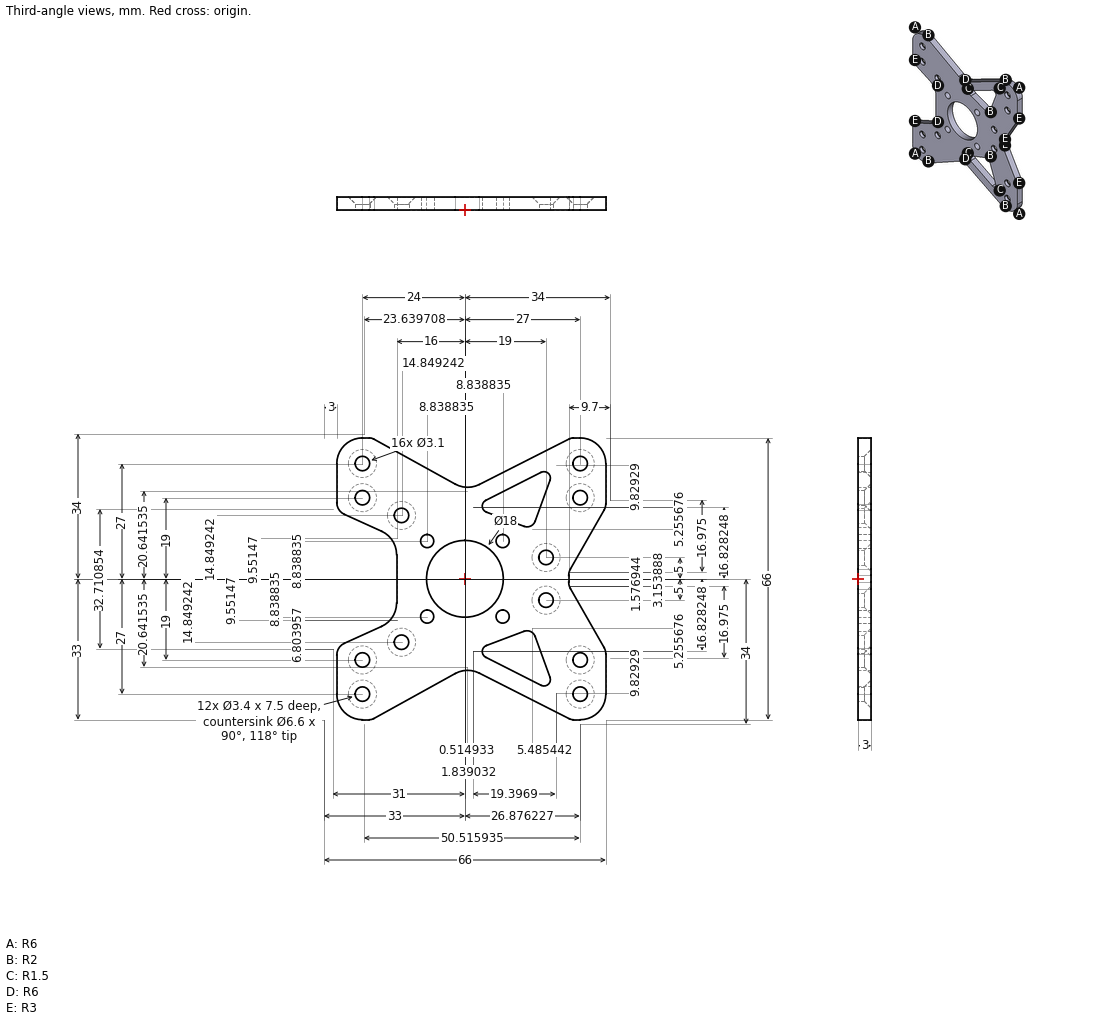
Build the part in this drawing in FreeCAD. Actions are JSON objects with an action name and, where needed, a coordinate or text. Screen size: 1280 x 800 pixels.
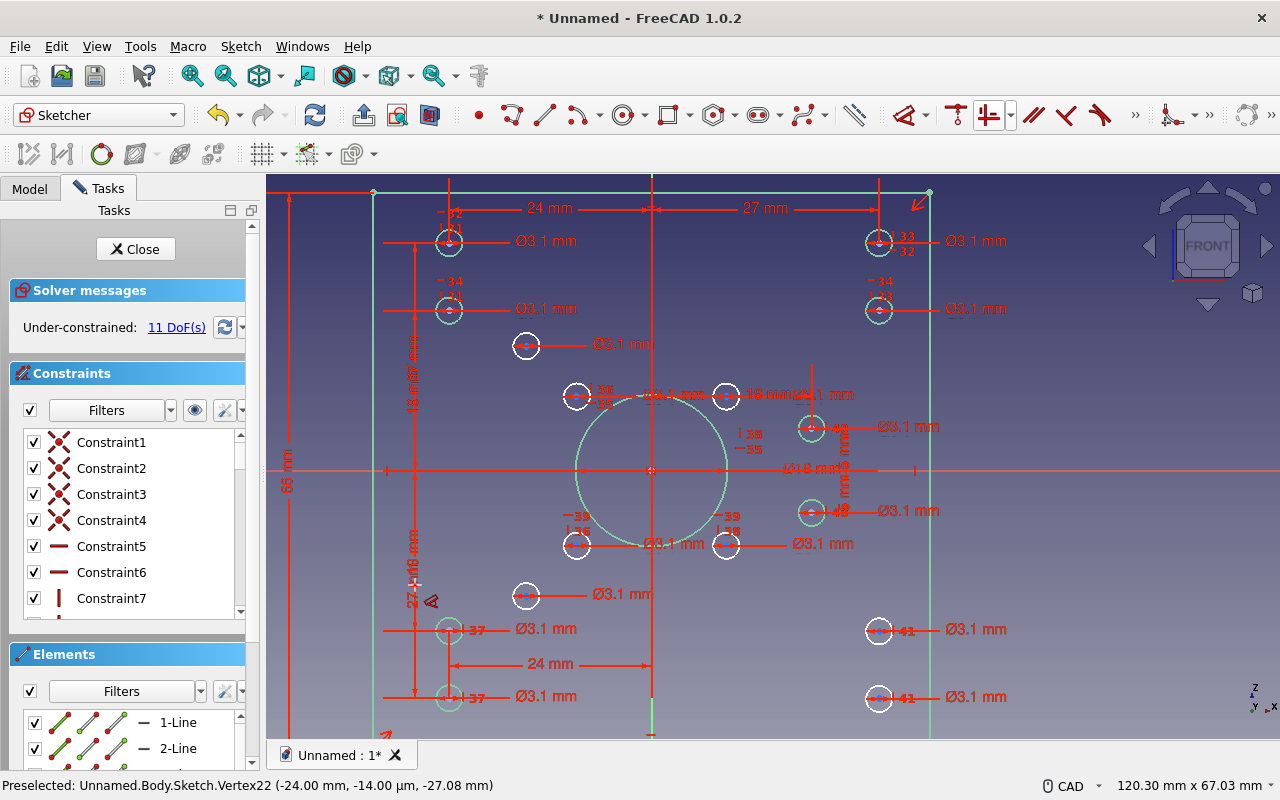
{"action": "left_click", "coordinate": [879, 631]}
{"action": "left_click", "coordinate": [765, 665]}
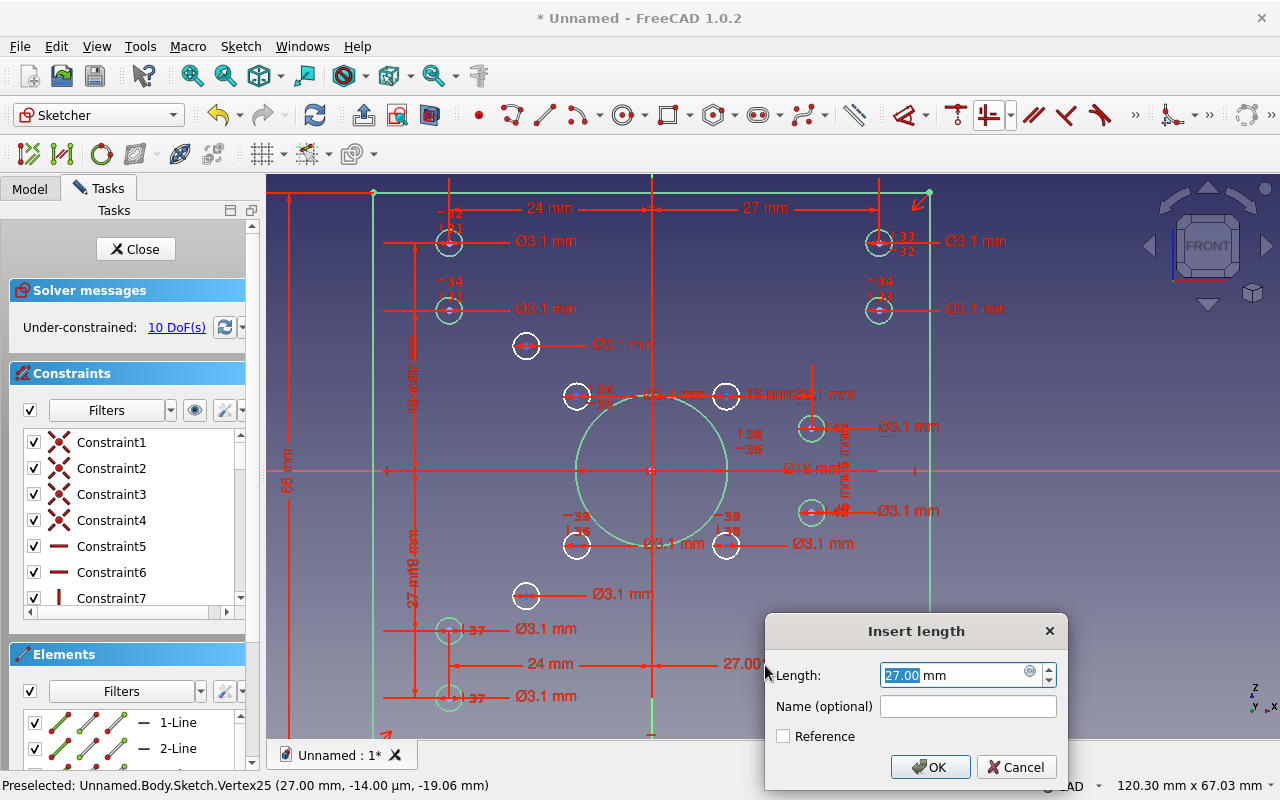
{"action": "type", "text": "27"}
{"action": "key", "text": "Return"}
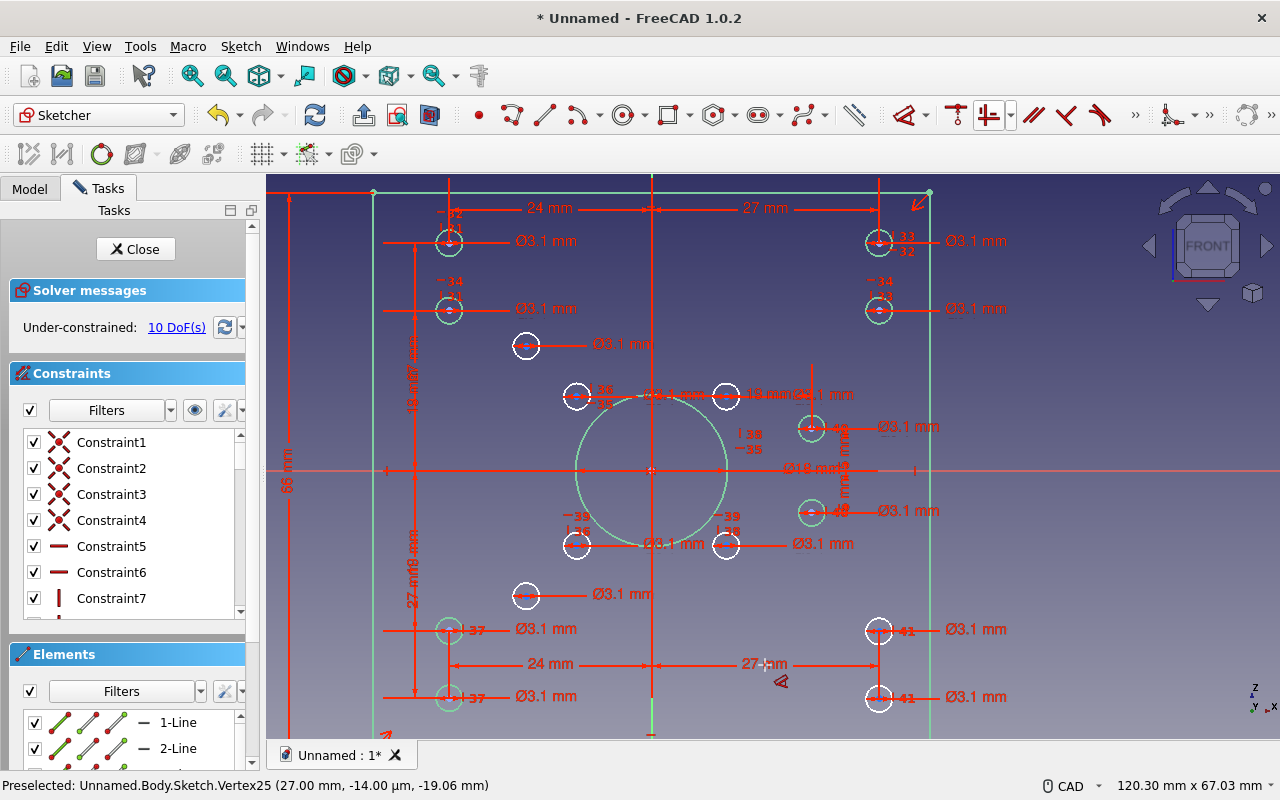
{"action": "left_click", "coordinate": [879, 631]}
{"action": "left_click", "coordinate": [913, 551]}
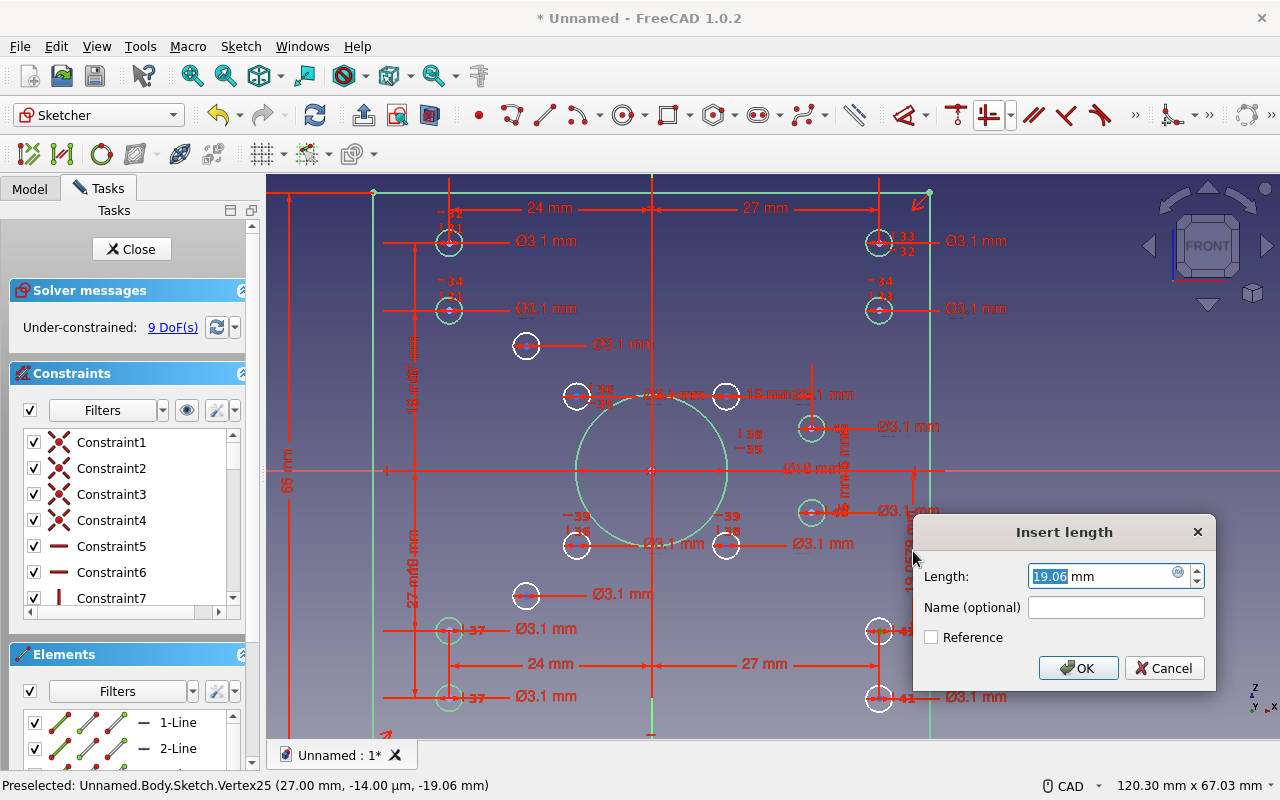
{"action": "type", "text": "19"}
{"action": "key", "text": "Return"}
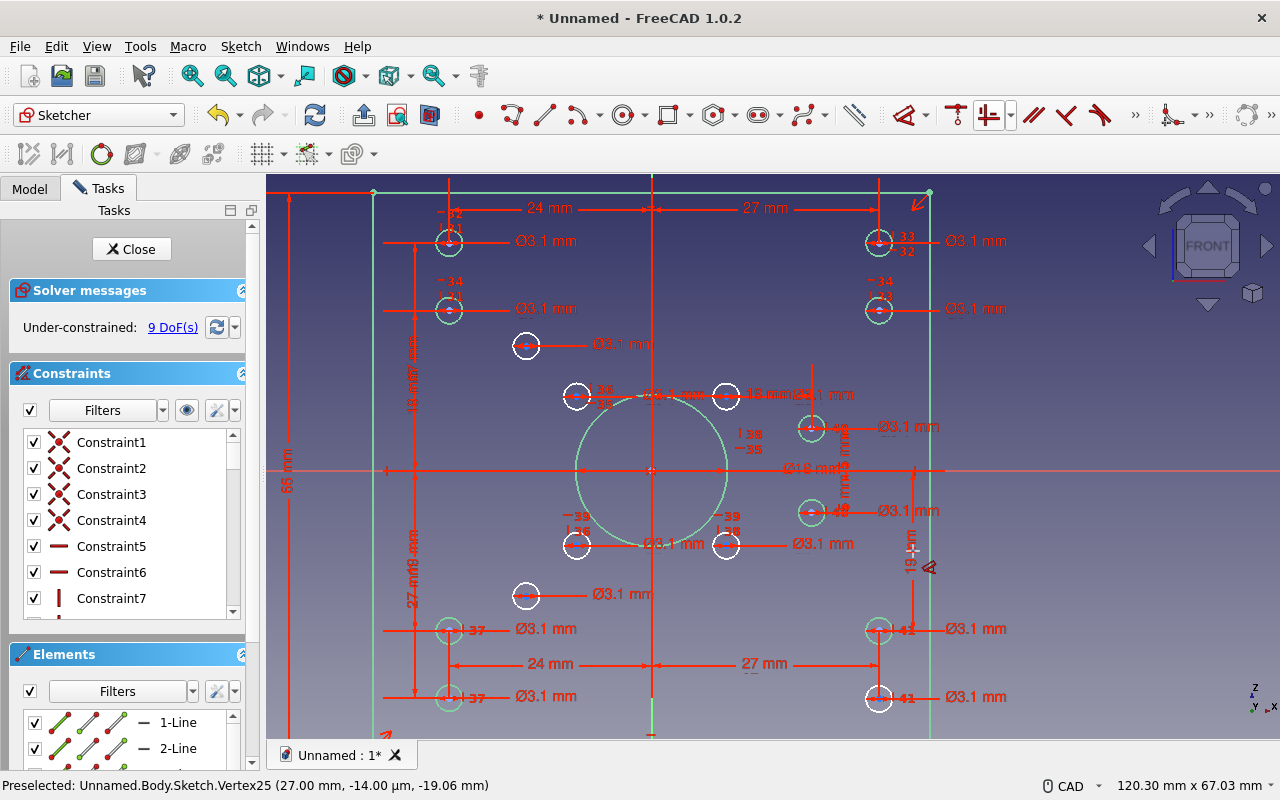
{"action": "left_click", "coordinate": [879, 699]}
{"action": "left_click", "coordinate": [913, 585]}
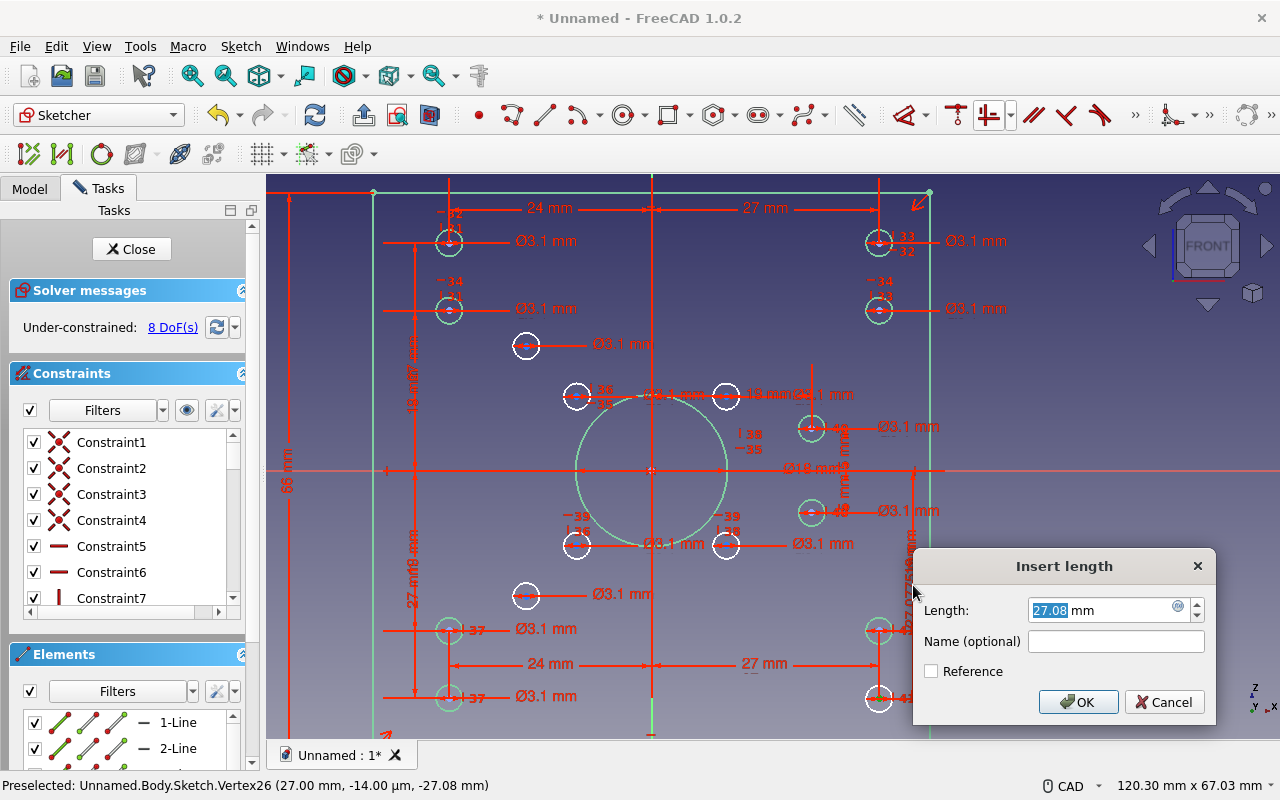
{"action": "type", "text": "27"}
{"action": "key", "text": "Return"}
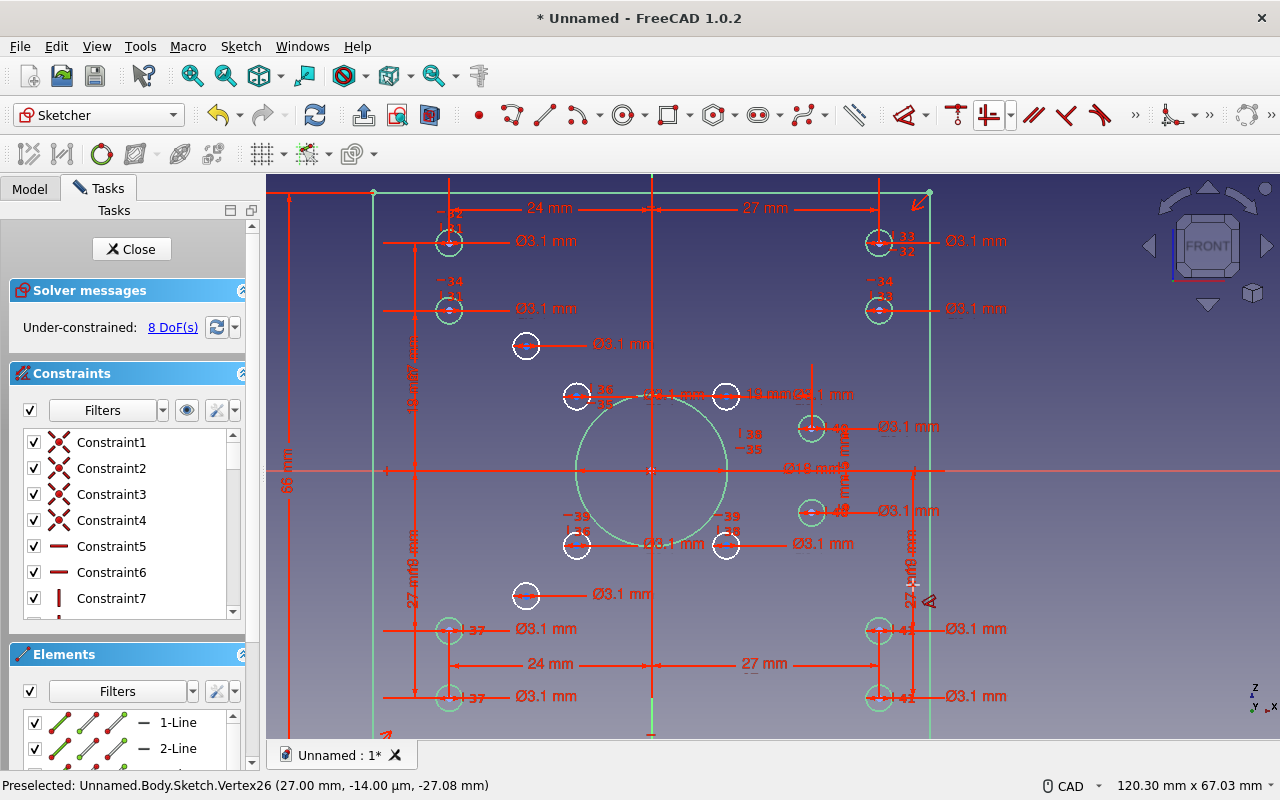
{"action": "left_click", "coordinate": [577, 397]}
{"action": "left_click", "coordinate": [614, 363]}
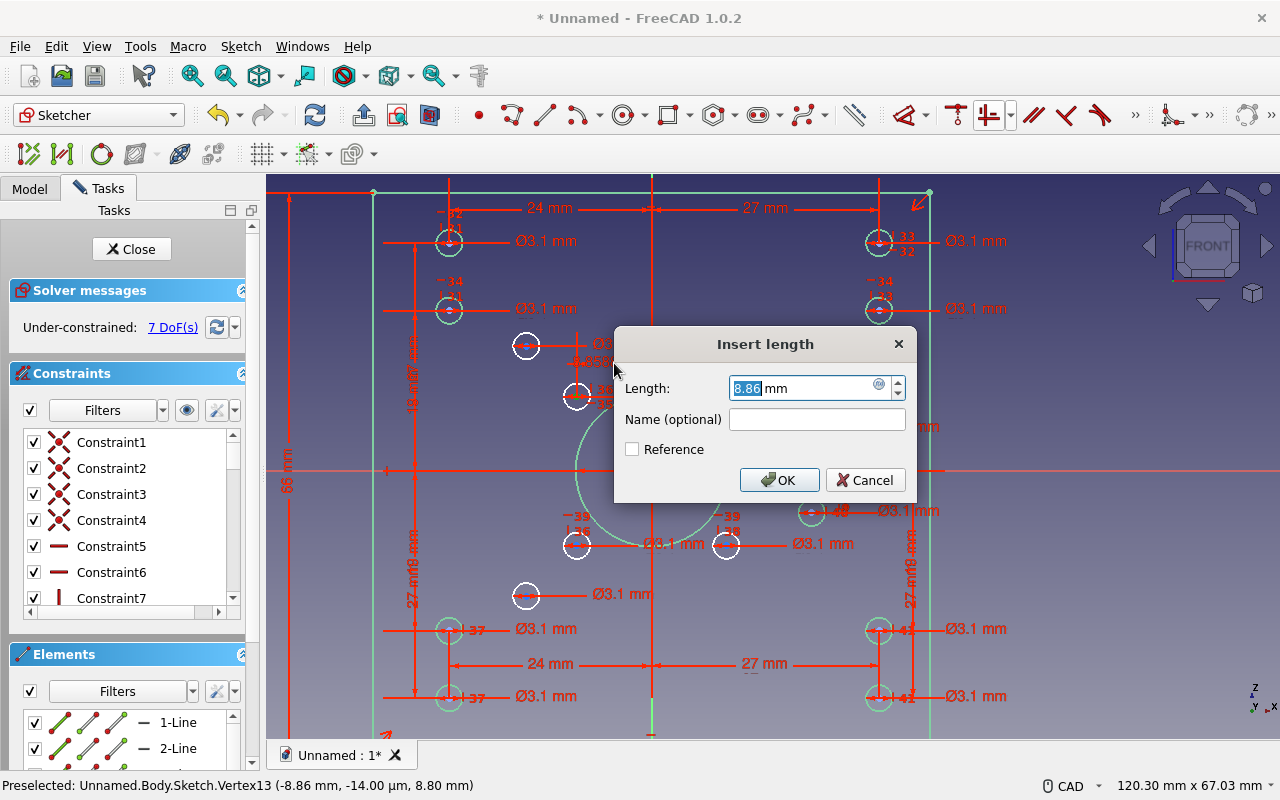
{"action": "type", "text": "8.838835"}
{"action": "key", "text": "Return"}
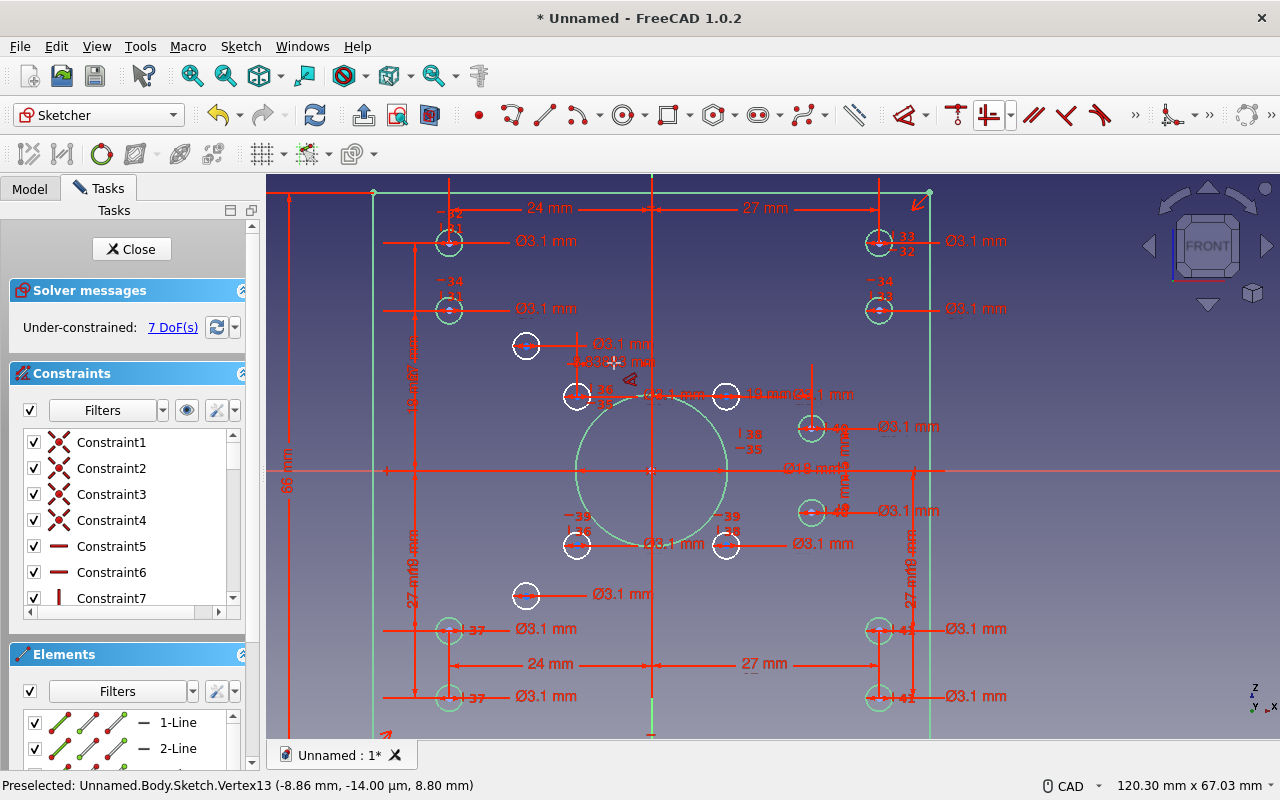
{"action": "left_click", "coordinate": [577, 397]}
{"action": "left_click", "coordinate": [543, 434]}